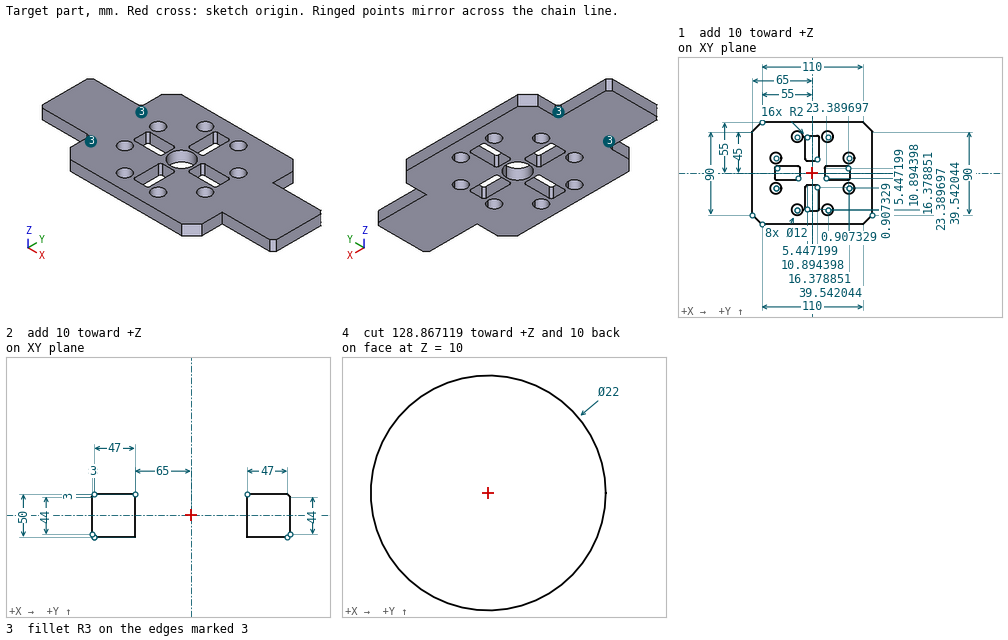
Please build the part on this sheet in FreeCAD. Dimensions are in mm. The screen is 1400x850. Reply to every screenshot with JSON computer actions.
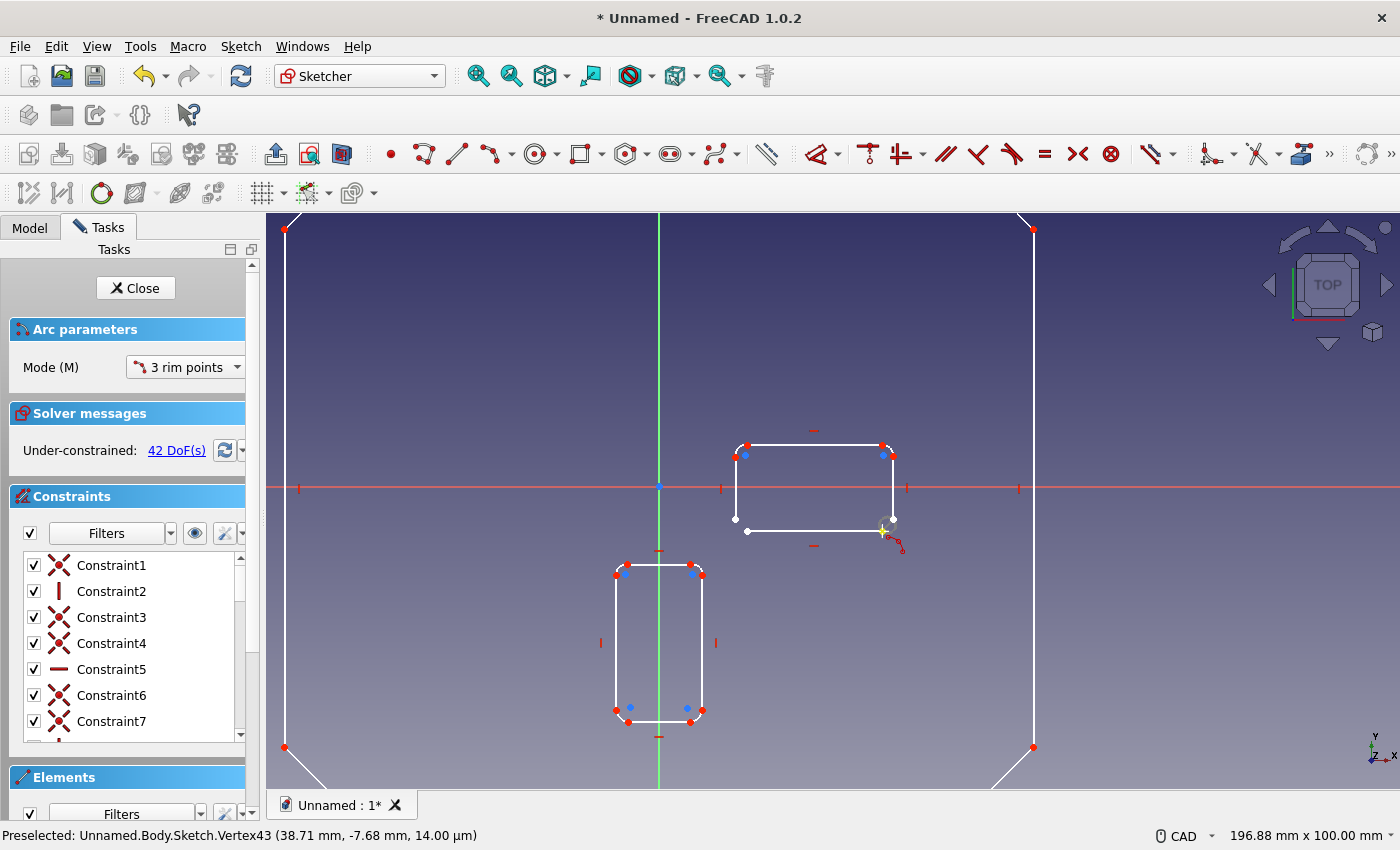
{"action": "scroll", "coordinate": [890, 526], "scroll_direction": "up", "scroll_amount": 8}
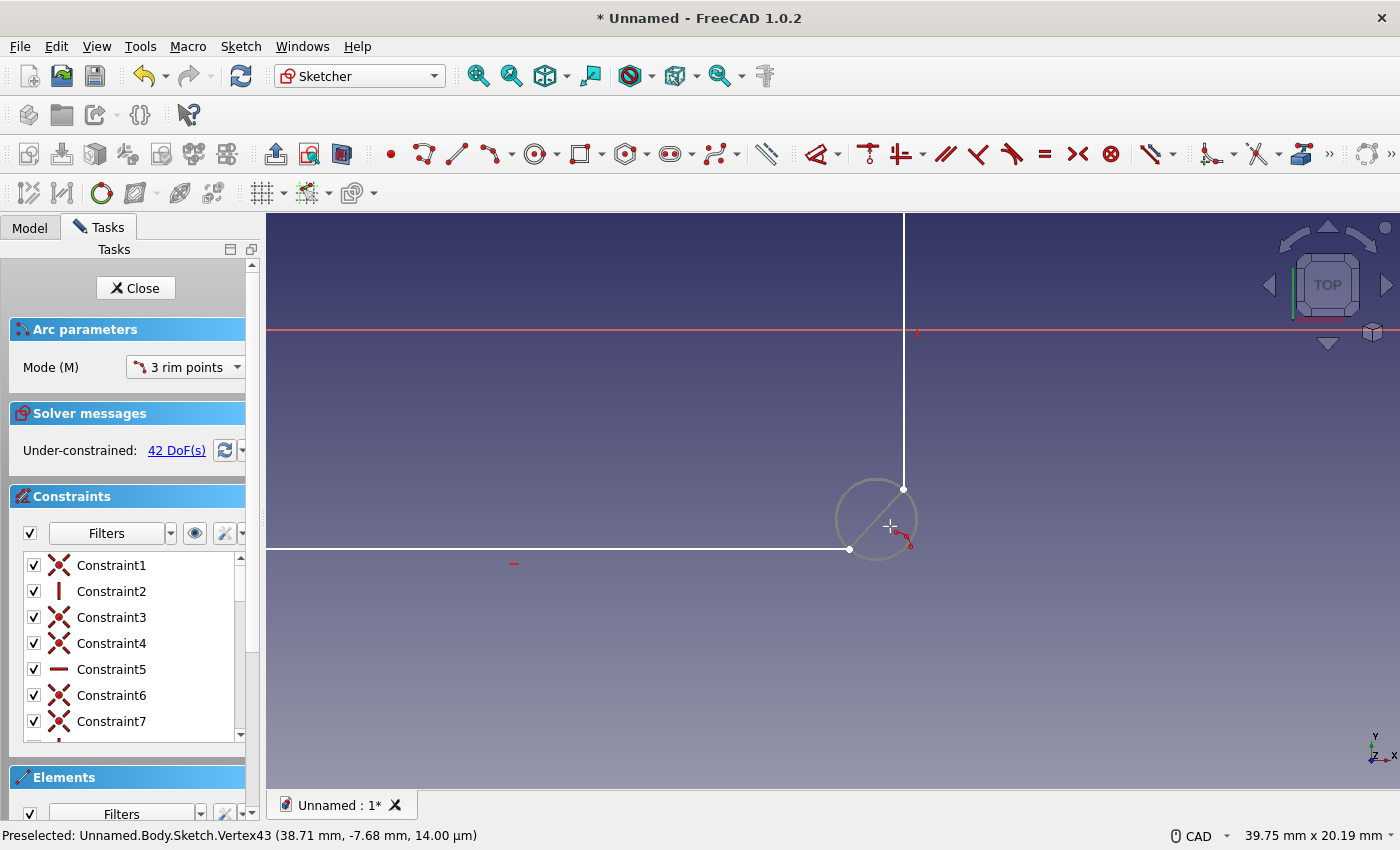
{"action": "left_click", "coordinate": [887, 526]}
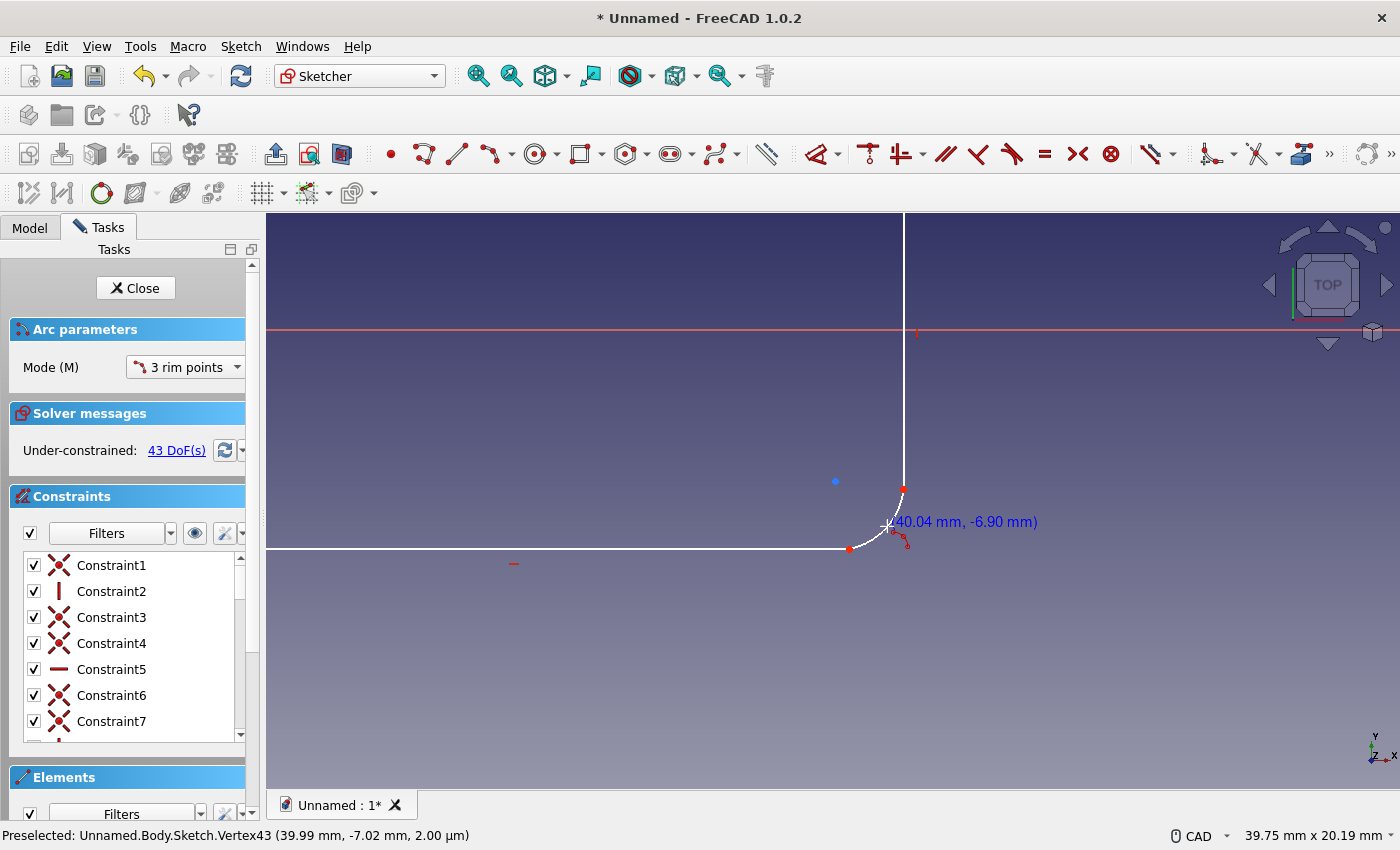
{"action": "scroll", "coordinate": [892, 522], "scroll_direction": "down", "scroll_amount": 11}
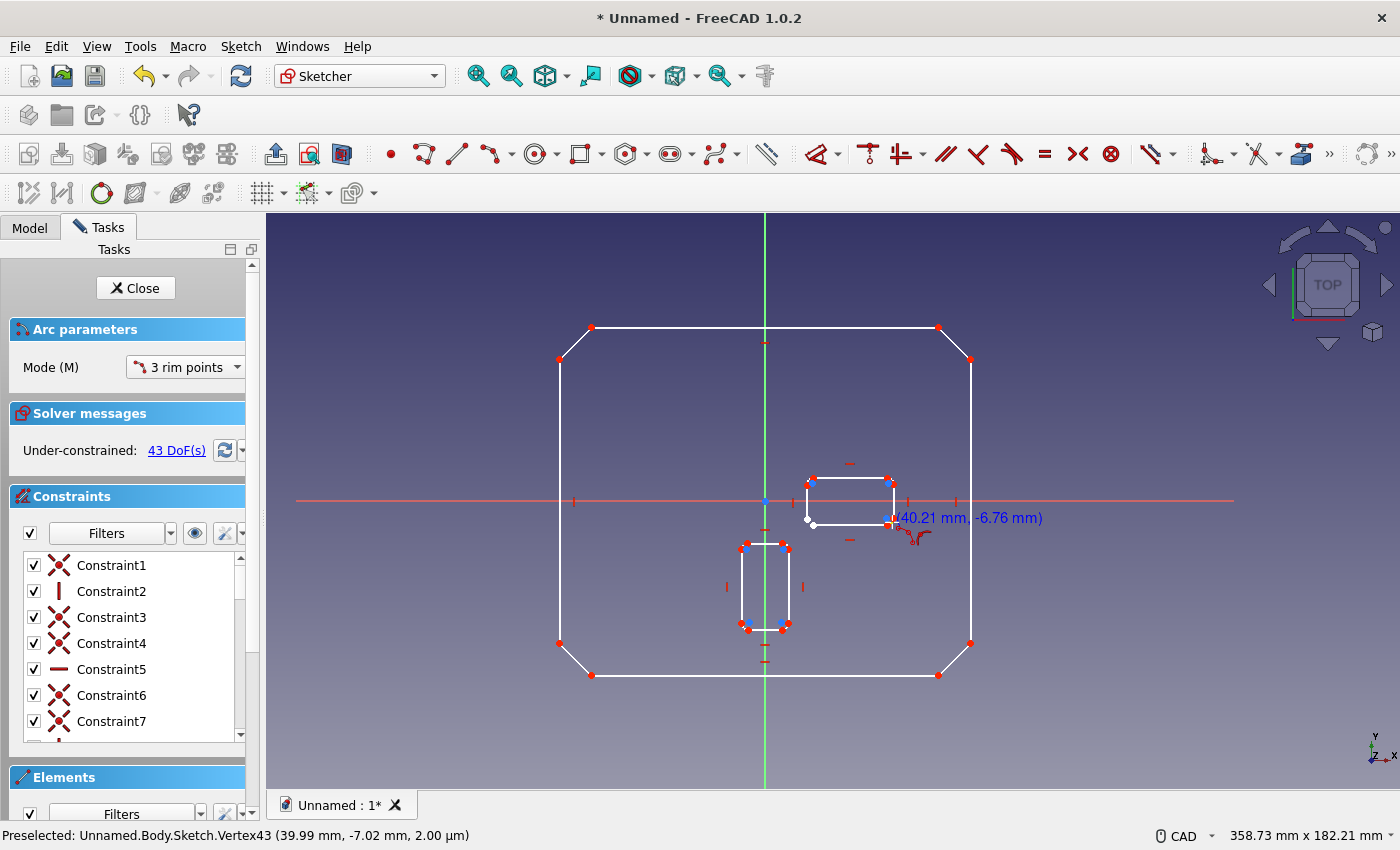
{"action": "scroll", "coordinate": [814, 525], "scroll_direction": "up", "scroll_amount": 3}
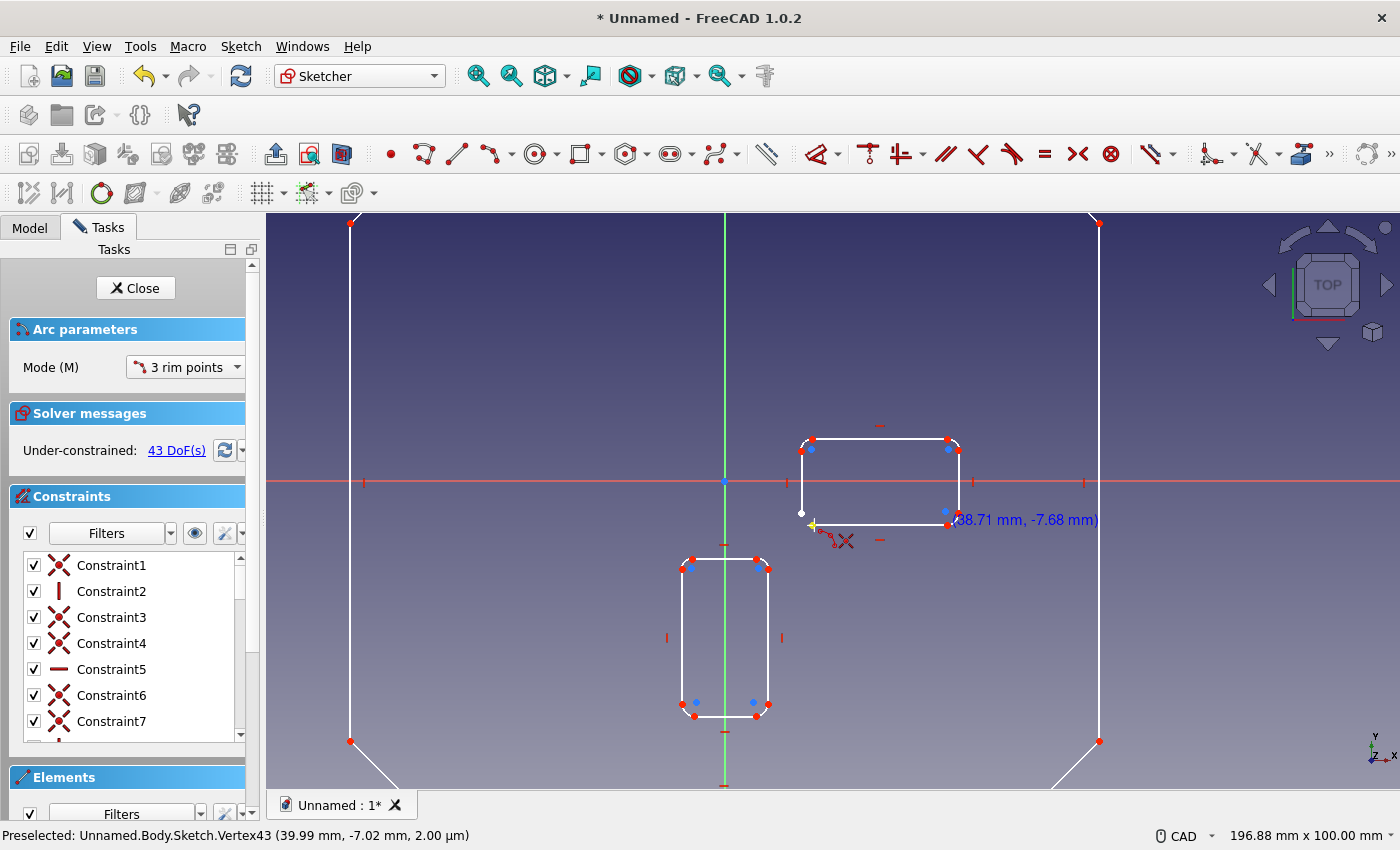
{"action": "left_click", "coordinate": [813, 525]}
{"action": "left_click", "coordinate": [802, 514]}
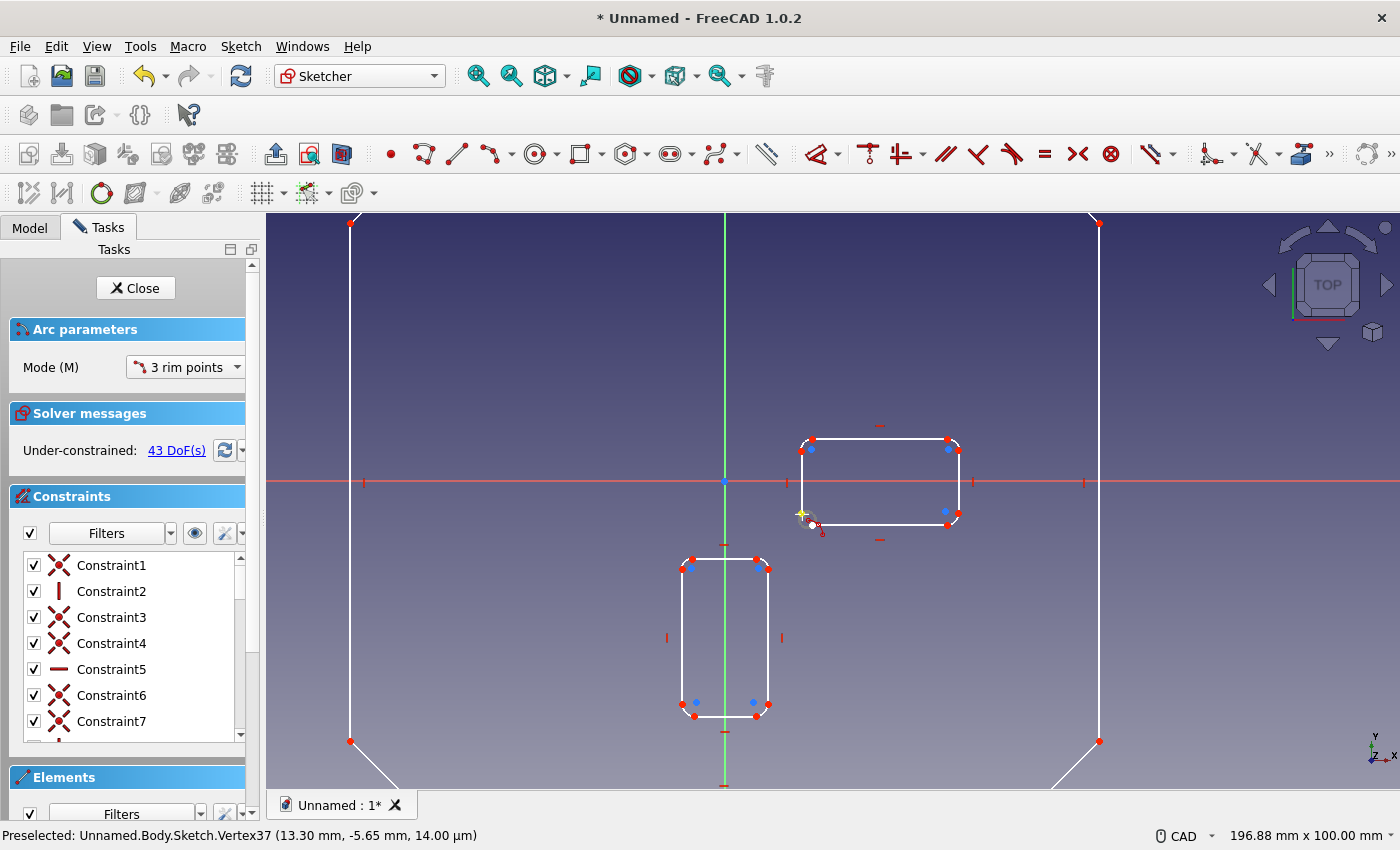
{"action": "scroll", "coordinate": [805, 521], "scroll_direction": "up", "scroll_amount": 8}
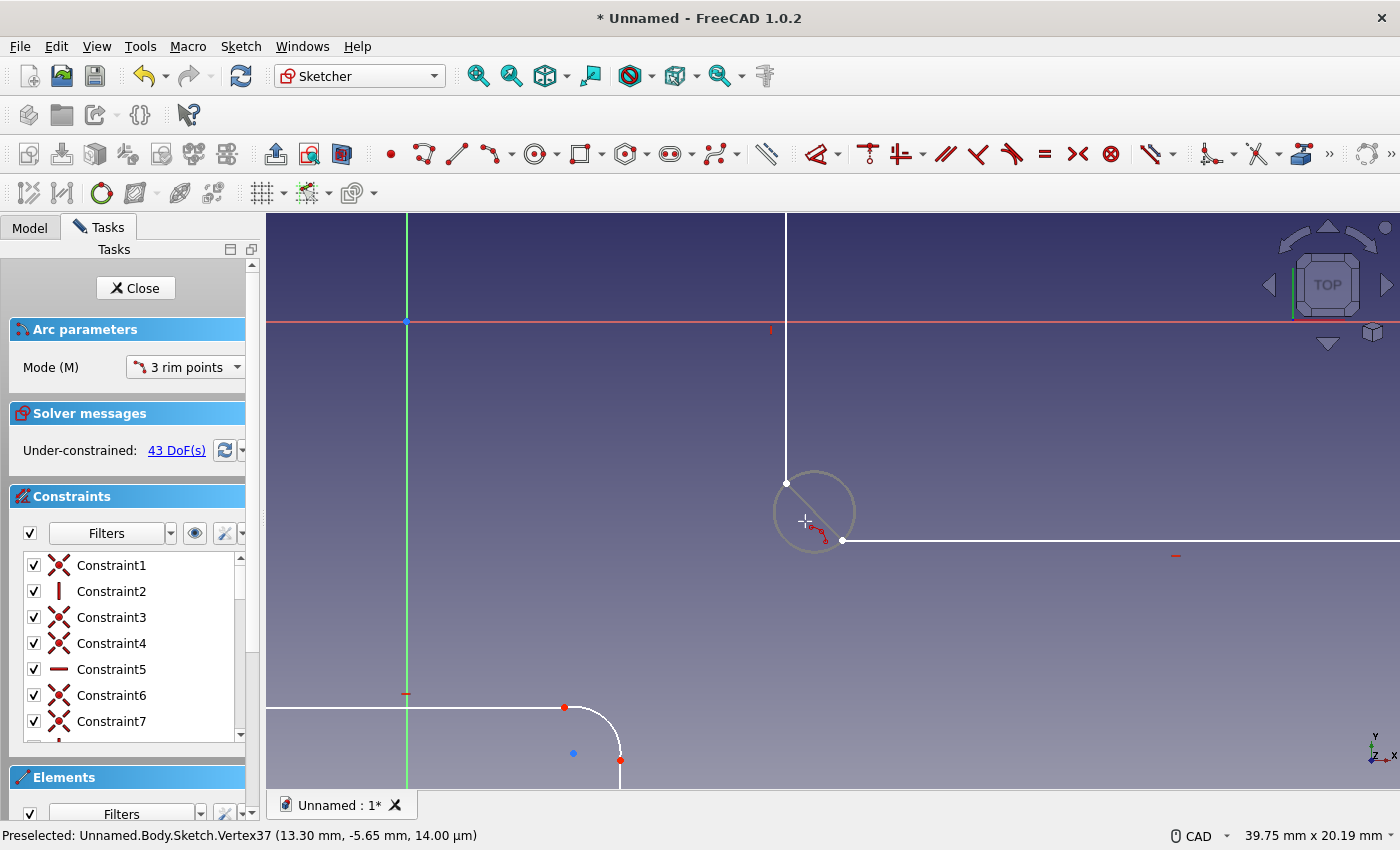
{"action": "left_click", "coordinate": [801, 518]}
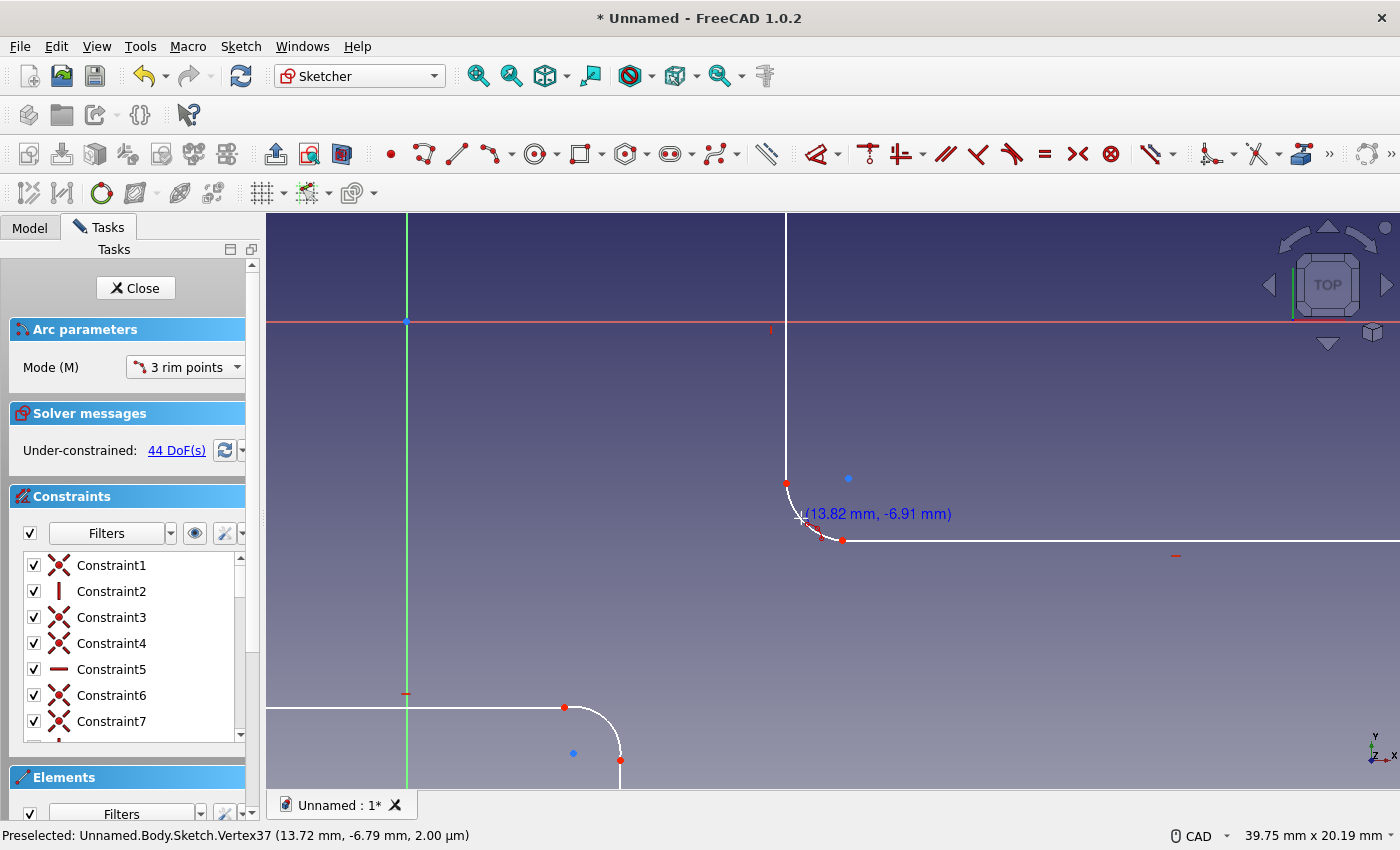
{"action": "left_click", "coordinate": [457, 154]}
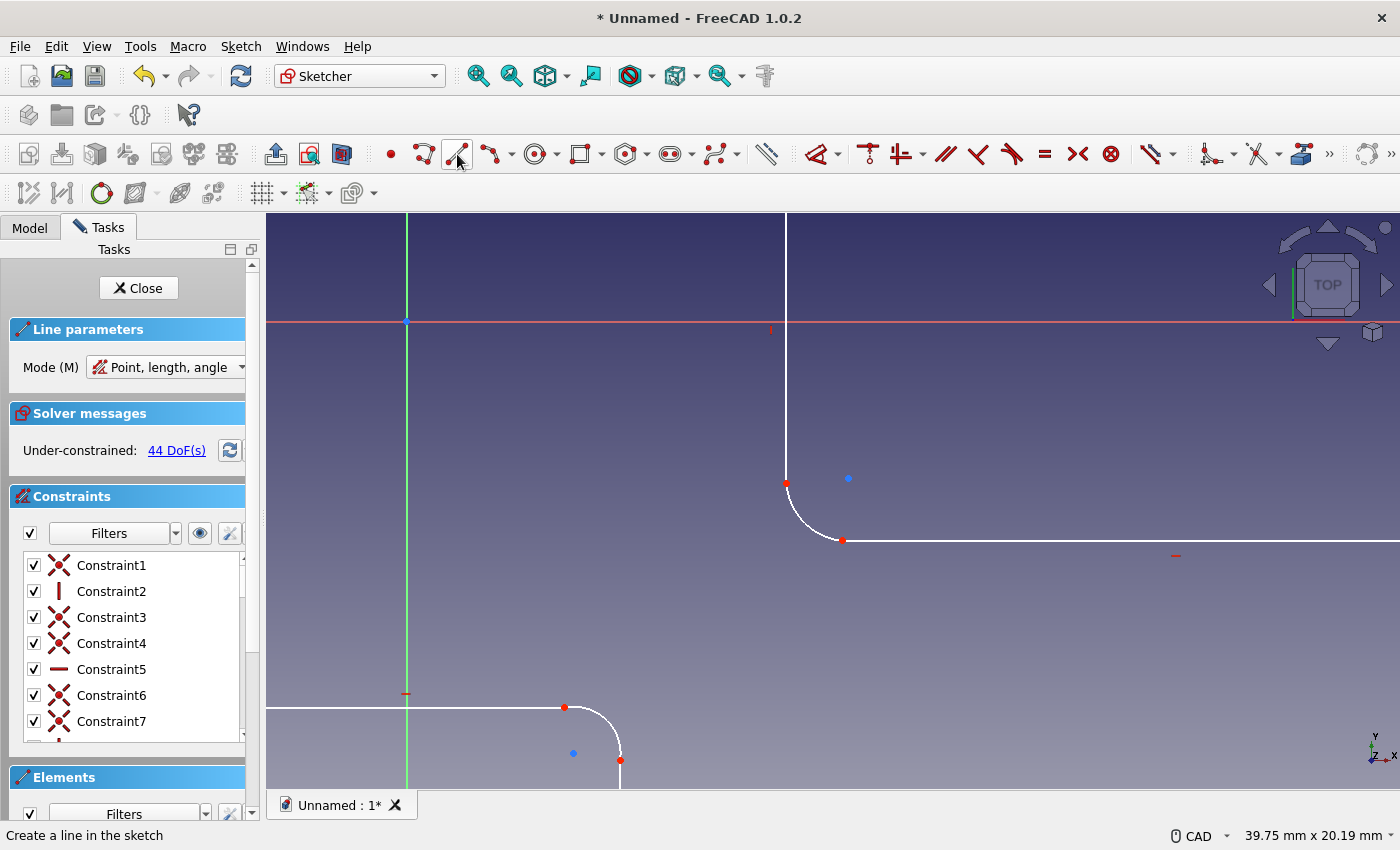
{"action": "scroll", "coordinate": [809, 523], "scroll_direction": "down", "scroll_amount": 11}